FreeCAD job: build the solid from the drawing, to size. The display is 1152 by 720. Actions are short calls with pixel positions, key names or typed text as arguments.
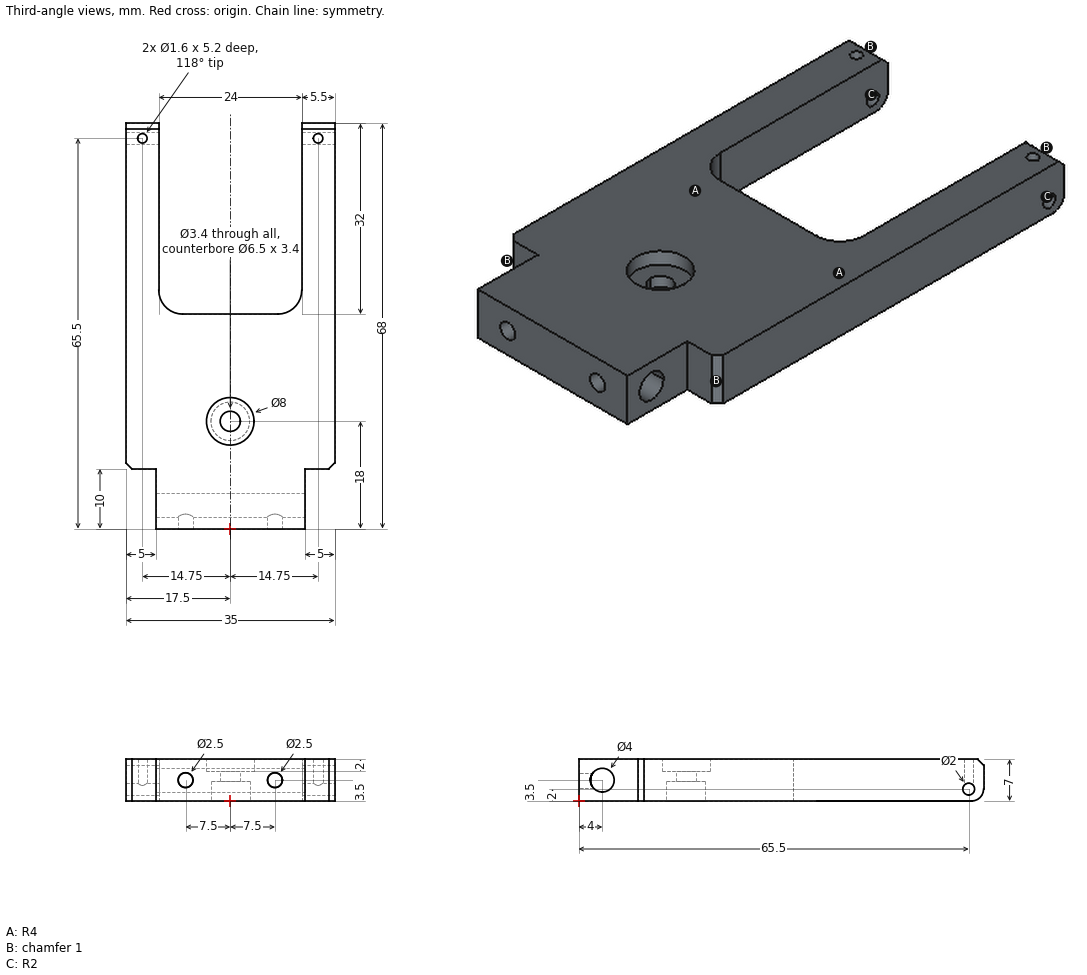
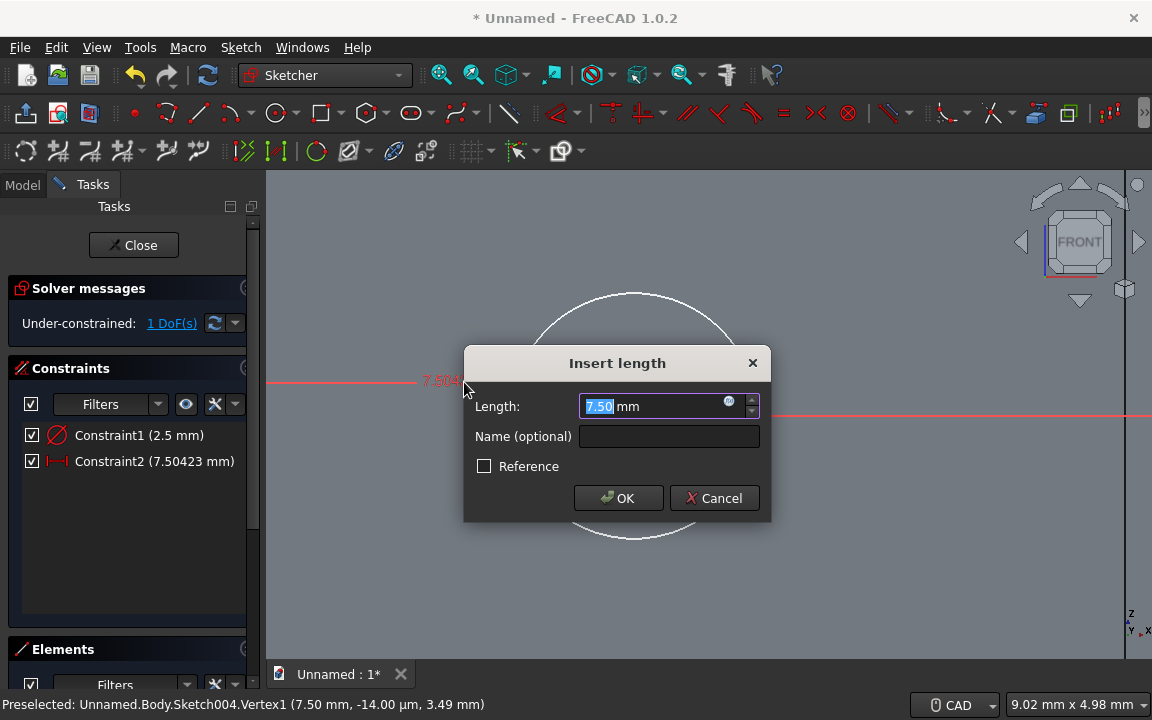
text(7.5)
key(Return)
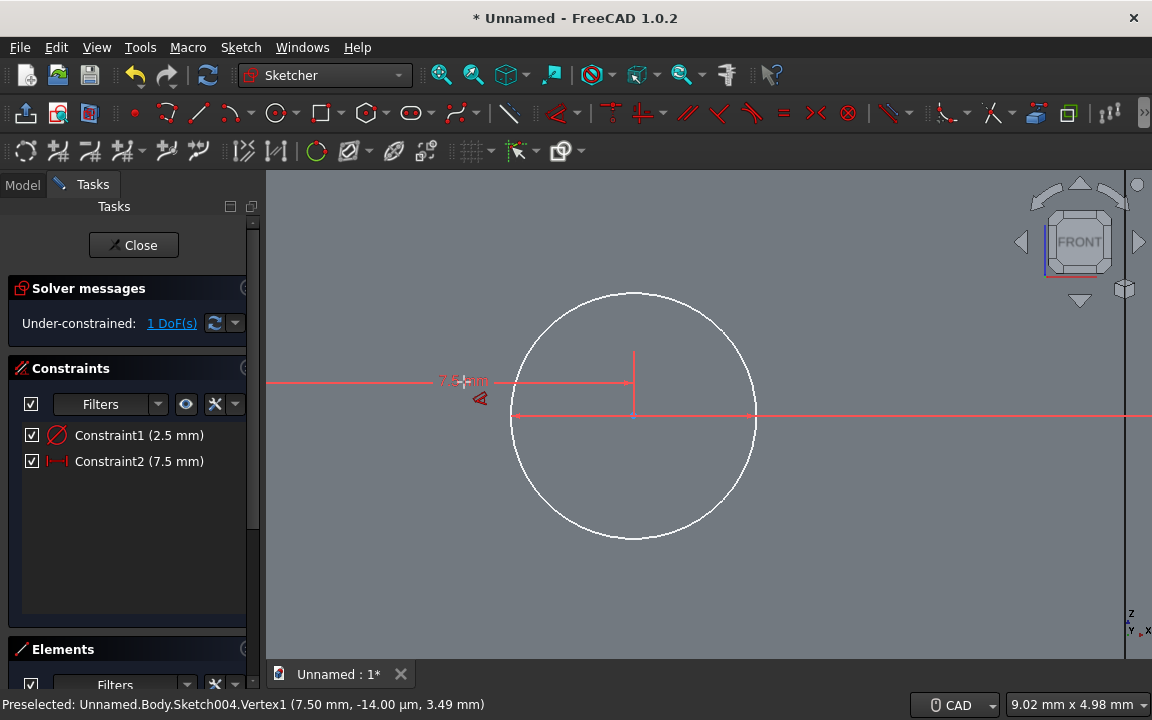
click(634, 416)
click(668, 474)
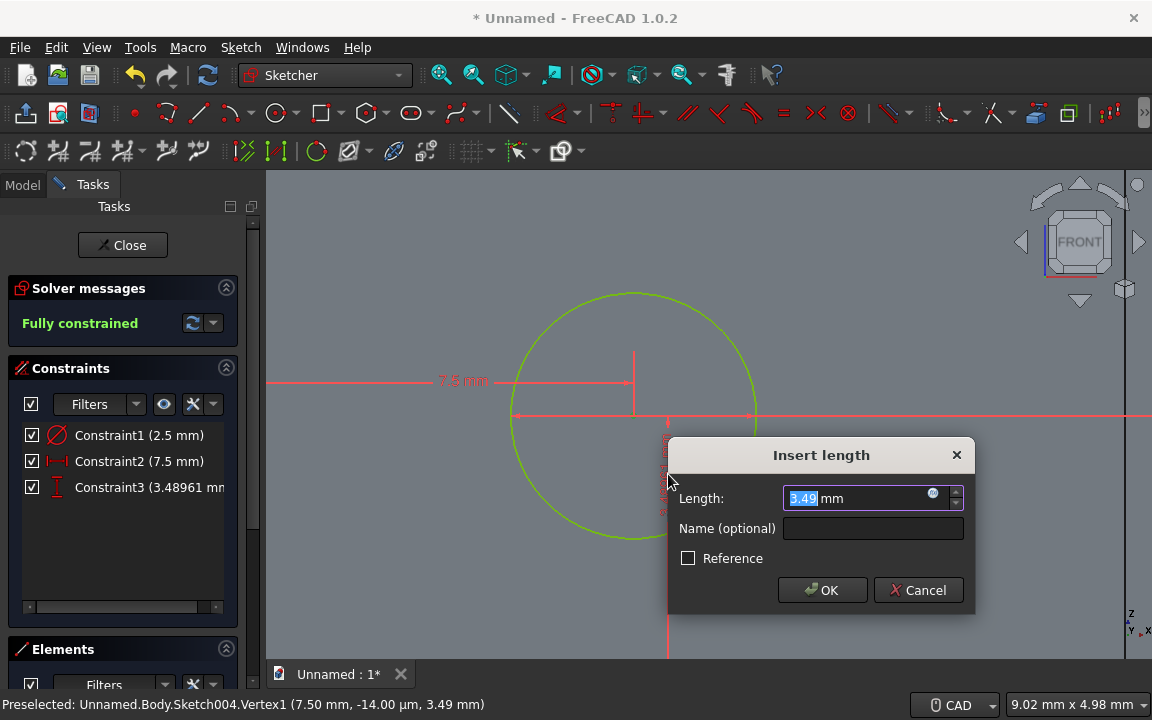
text(3.5)
key(Return)
key(Escape)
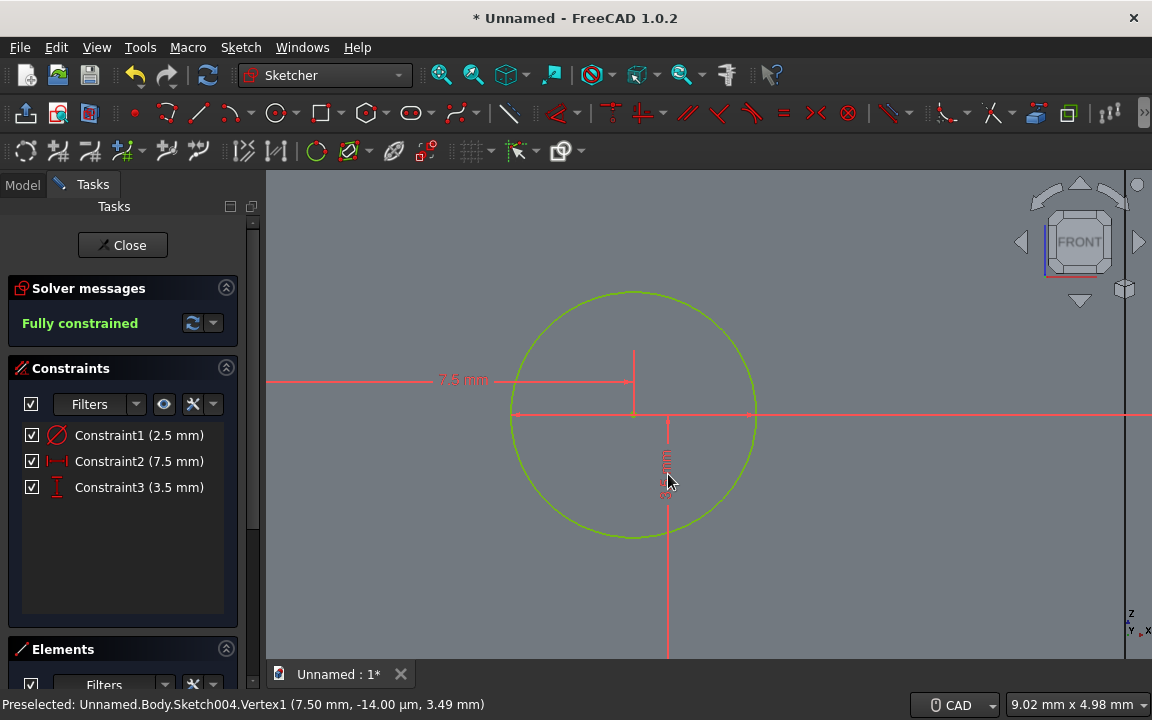
click(123, 245)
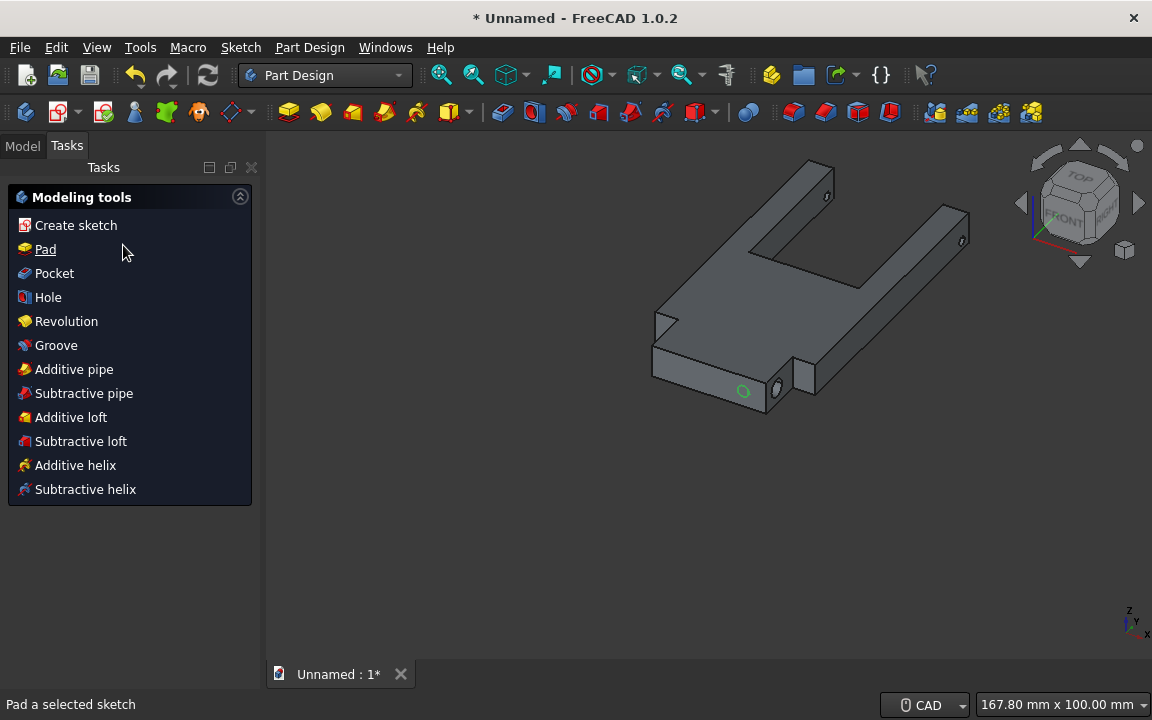
click(504, 112)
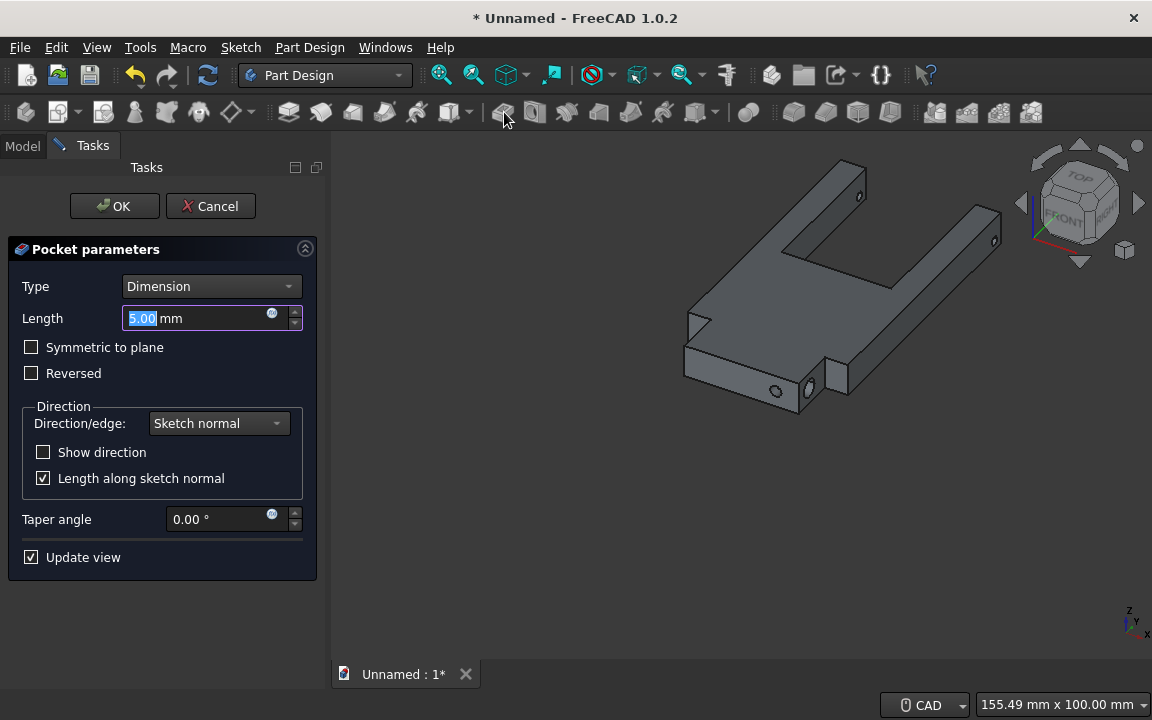
click(212, 286)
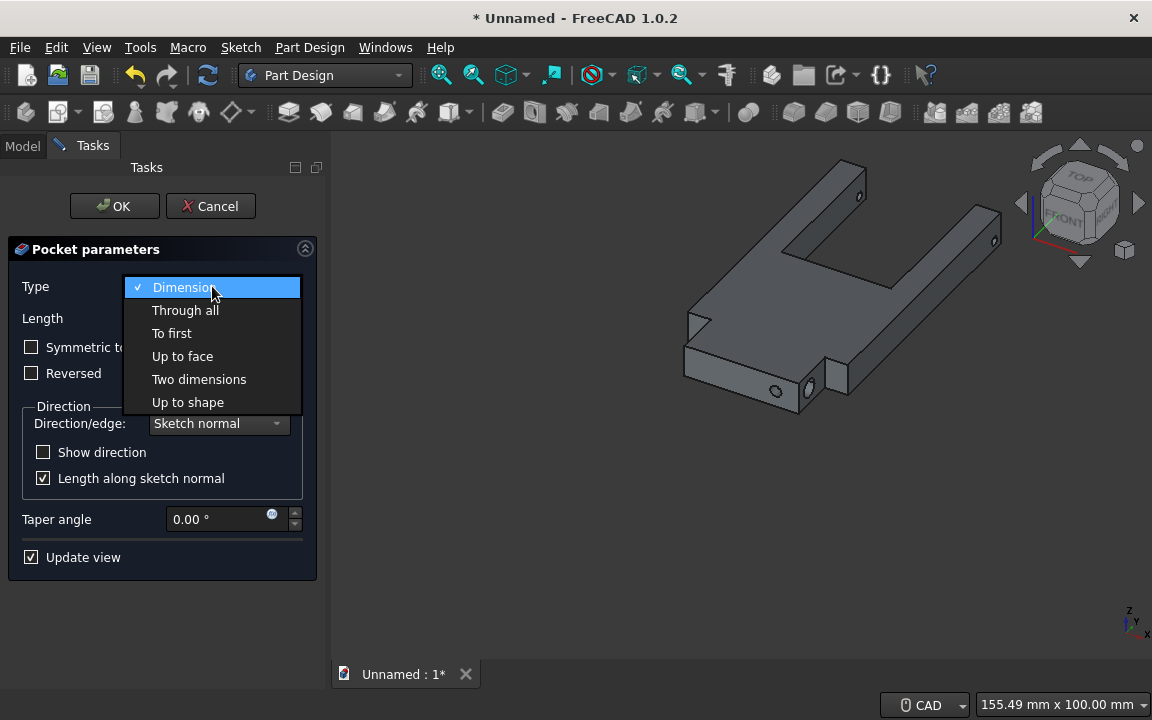
click(212, 334)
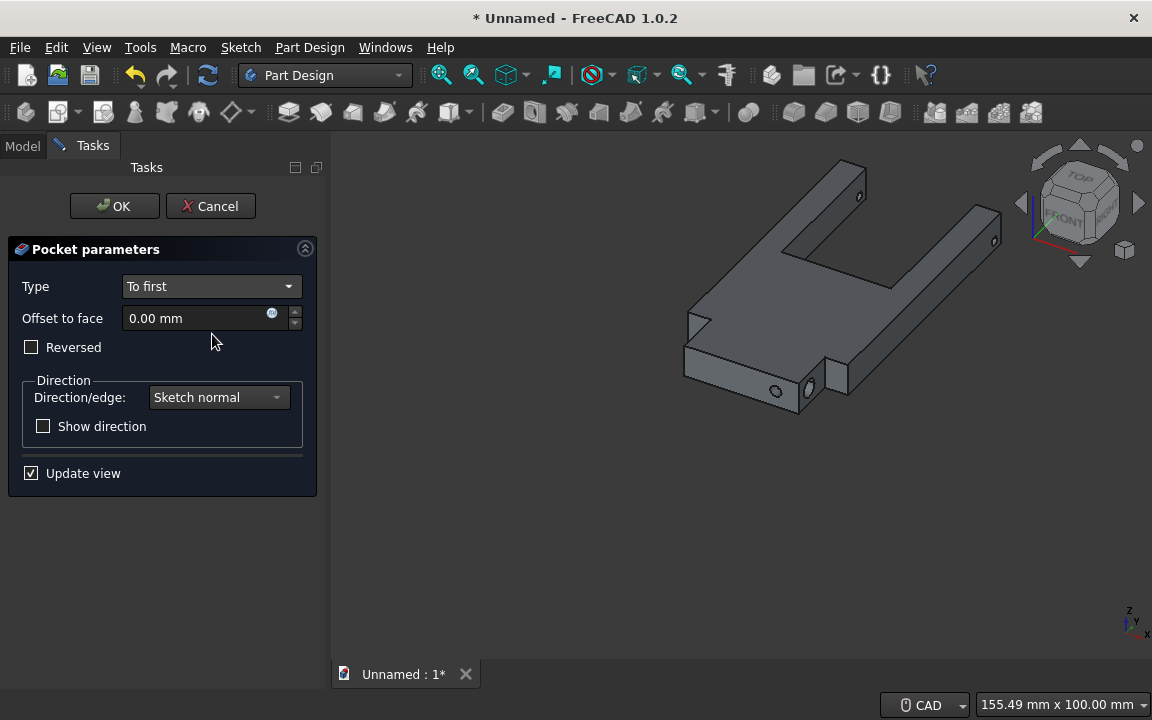
click(115, 206)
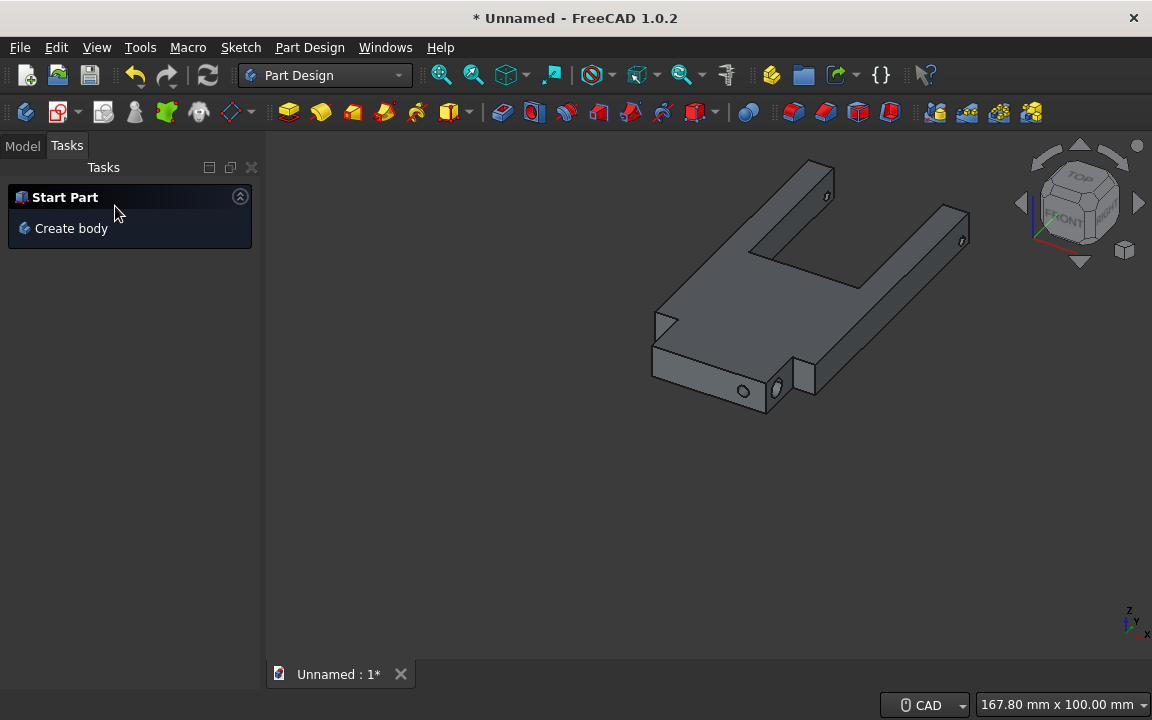
click(709, 379)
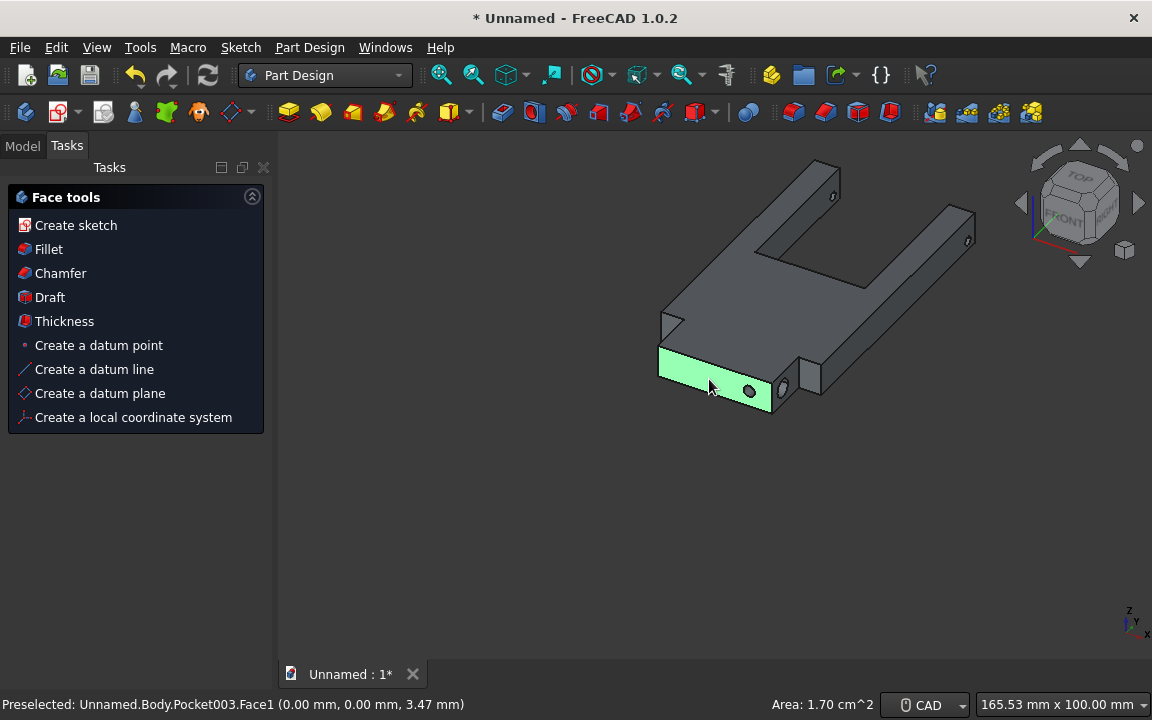
click(58, 112)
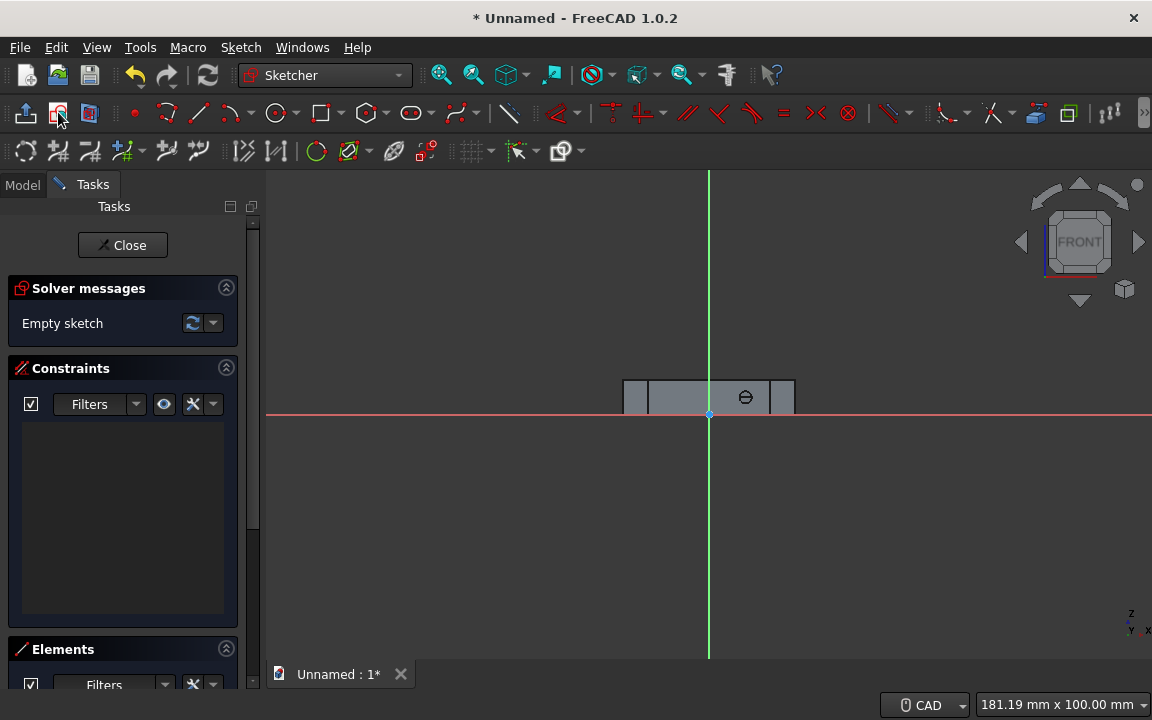
scroll(674, 396, up, 15)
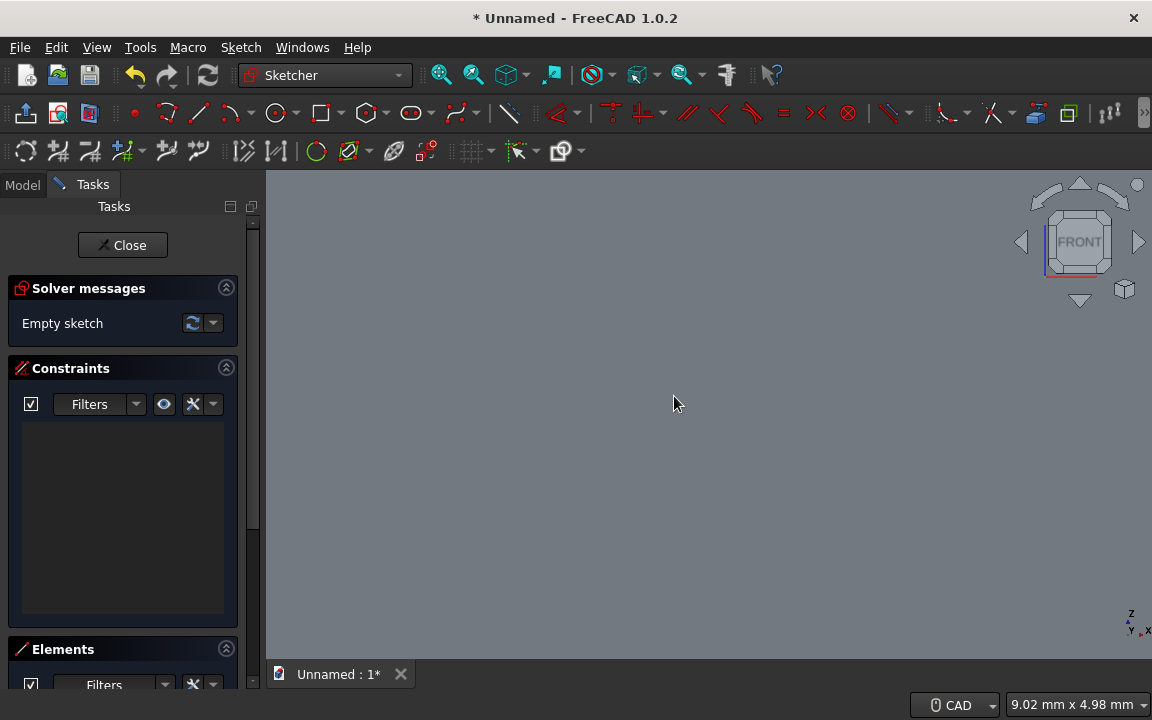
key(g)
key(c)